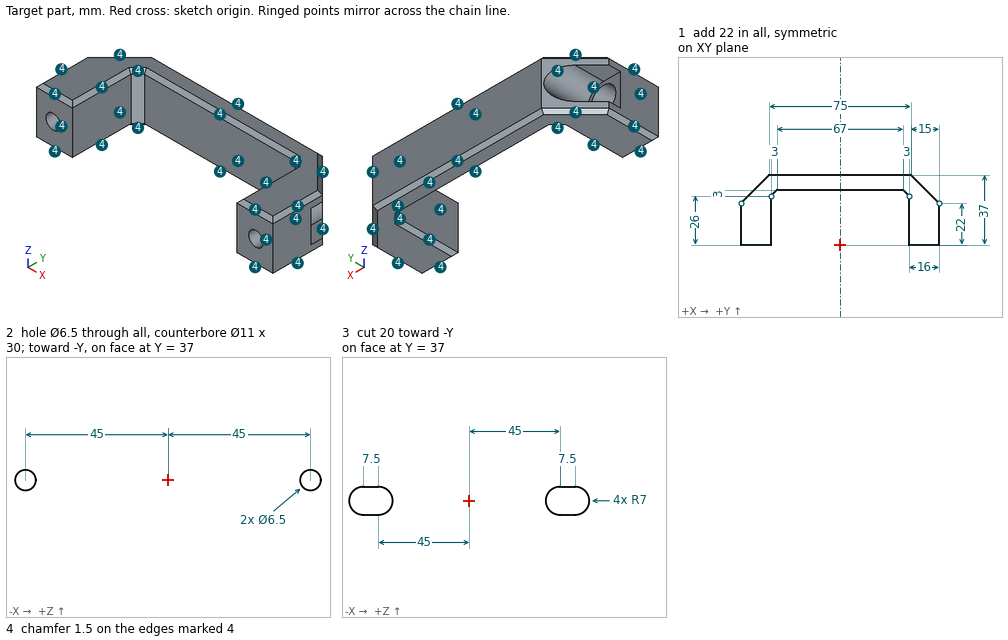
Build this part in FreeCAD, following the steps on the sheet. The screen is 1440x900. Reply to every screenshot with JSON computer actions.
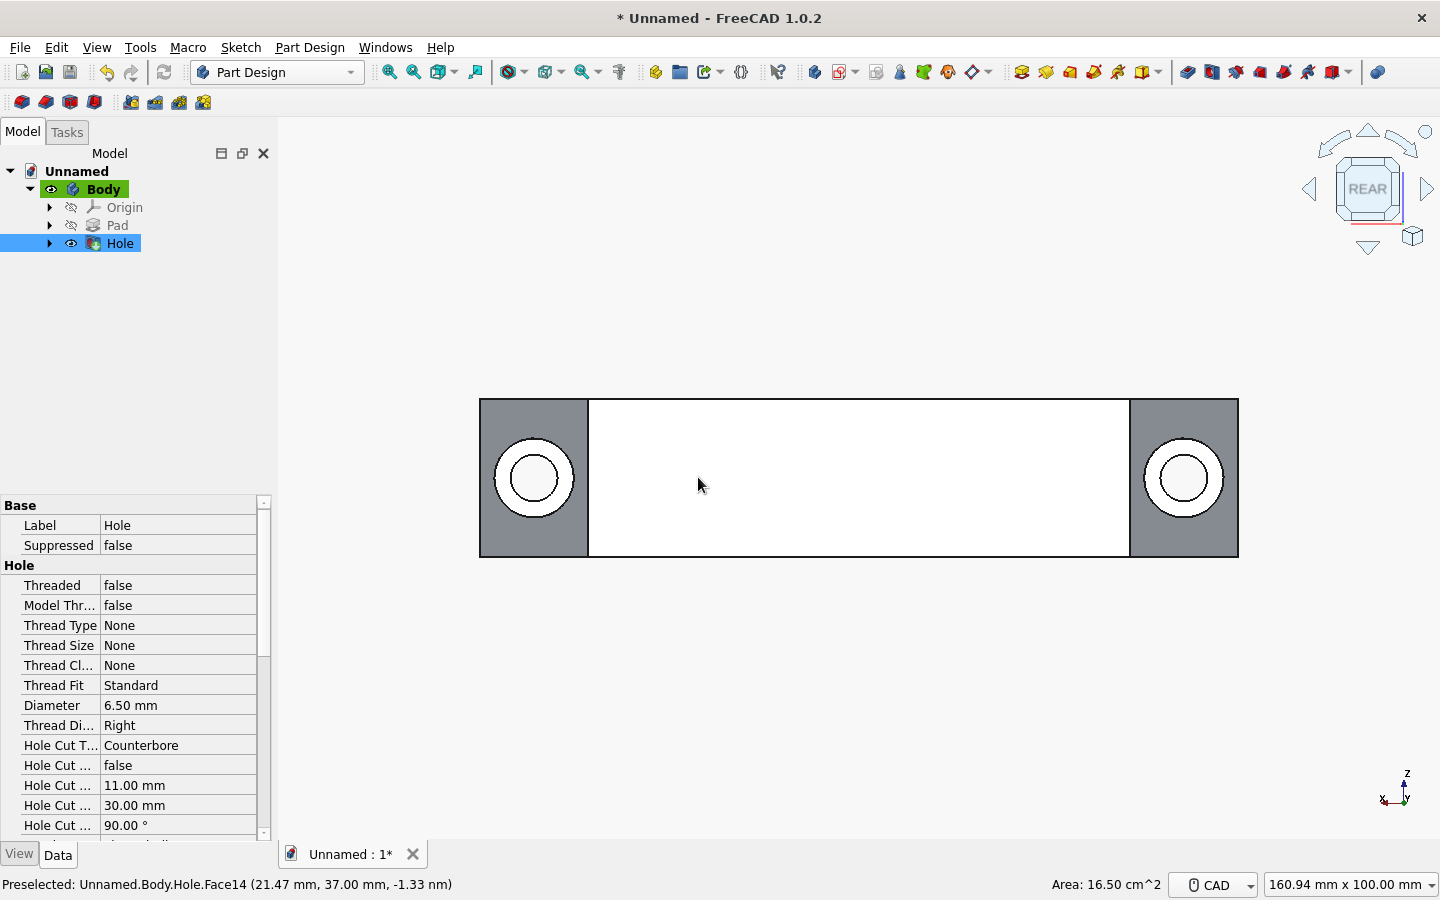
{"action": "left_click", "coordinate": [840, 72]}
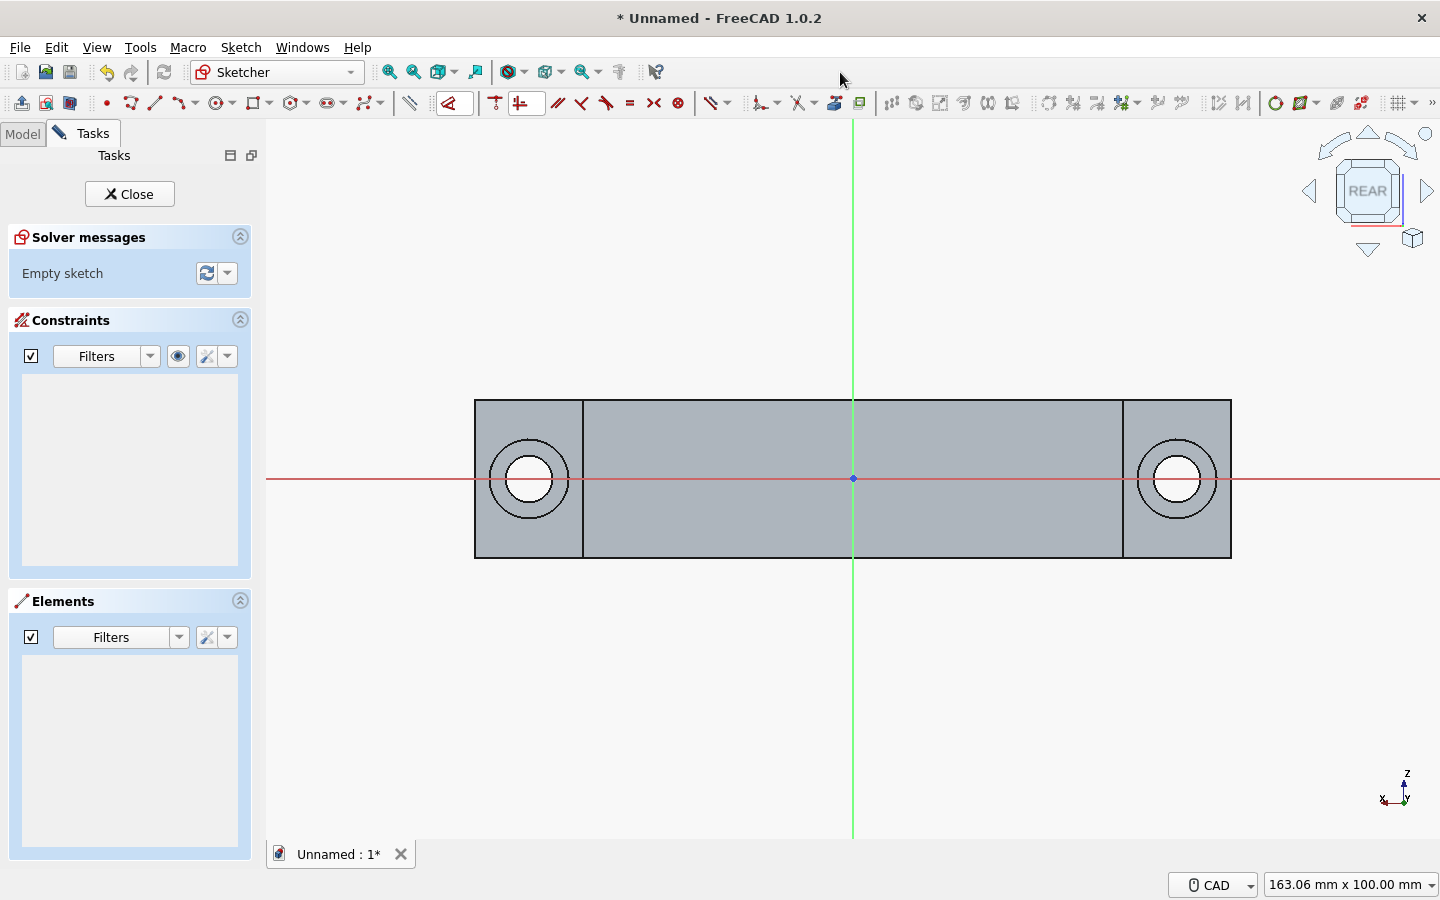
{"action": "scroll", "coordinate": [475, 479], "scroll_direction": "down", "scroll_amount": 1}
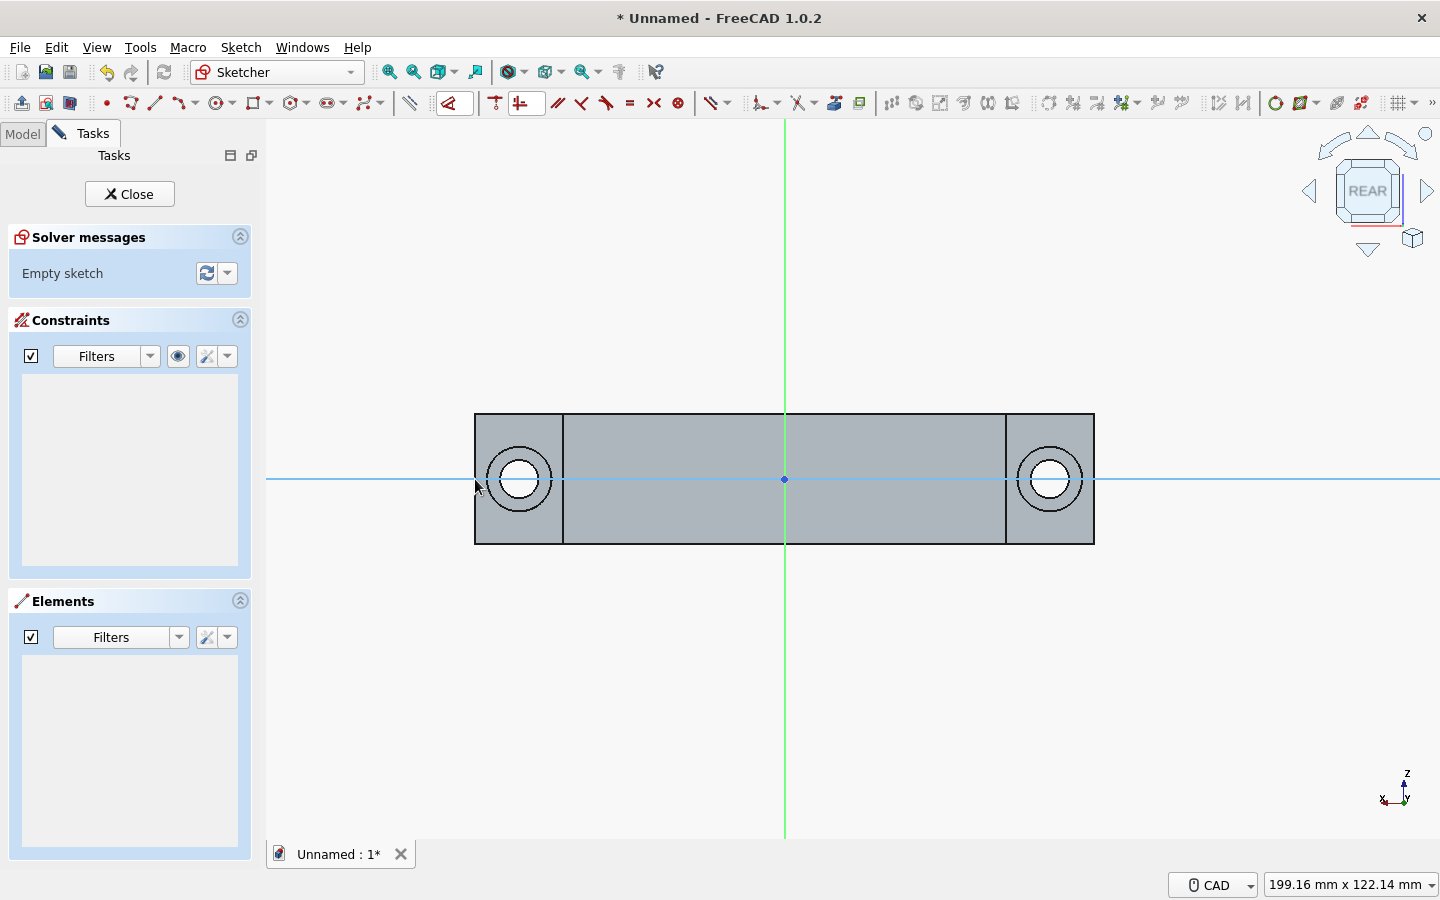
{"action": "left_click", "coordinate": [328, 104]}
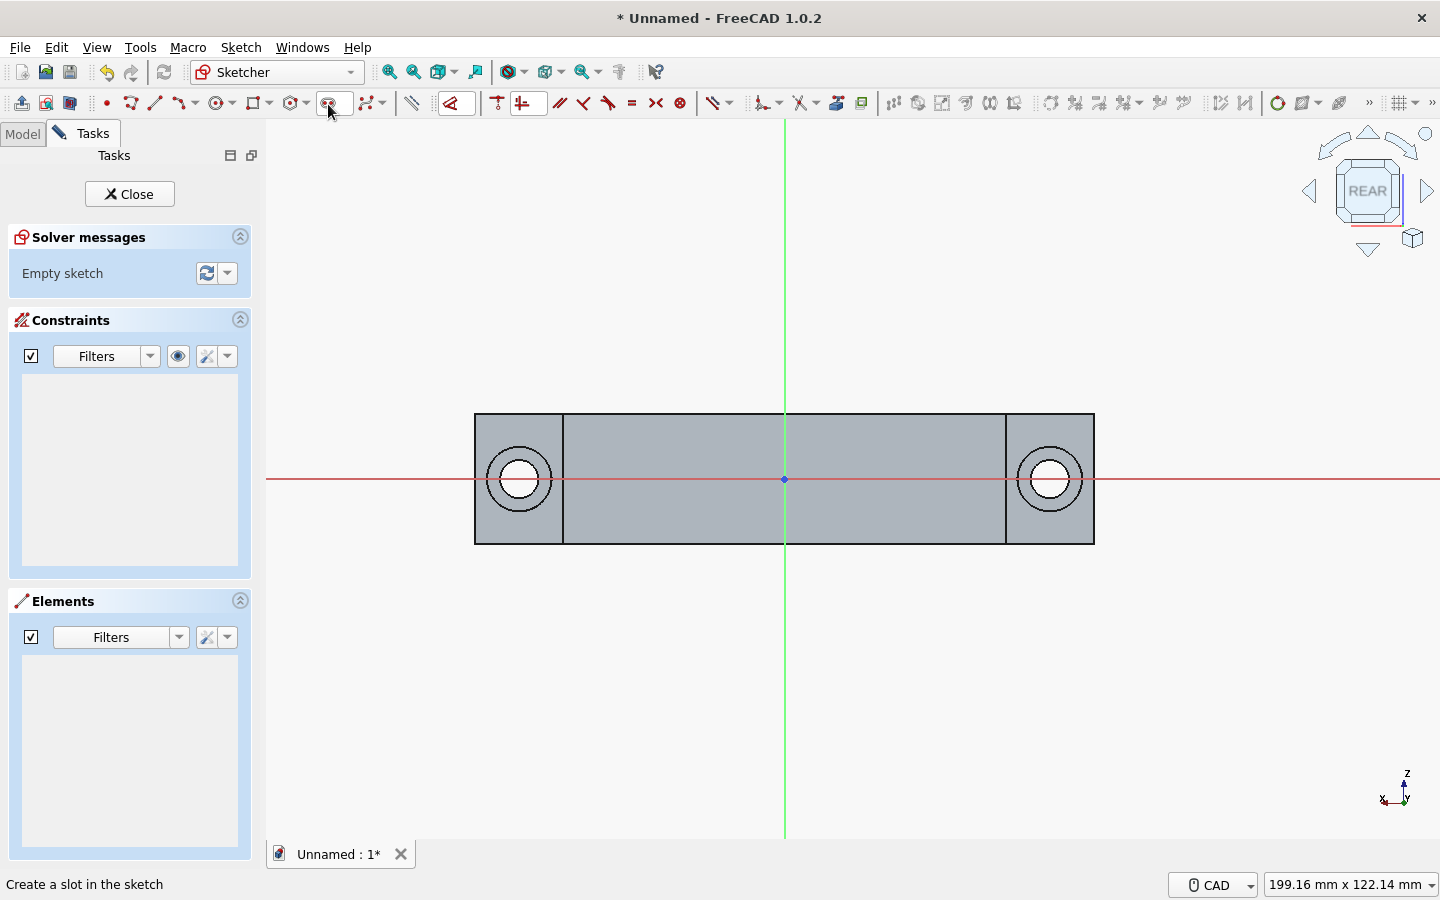
{"action": "left_click", "coordinate": [1050, 479]}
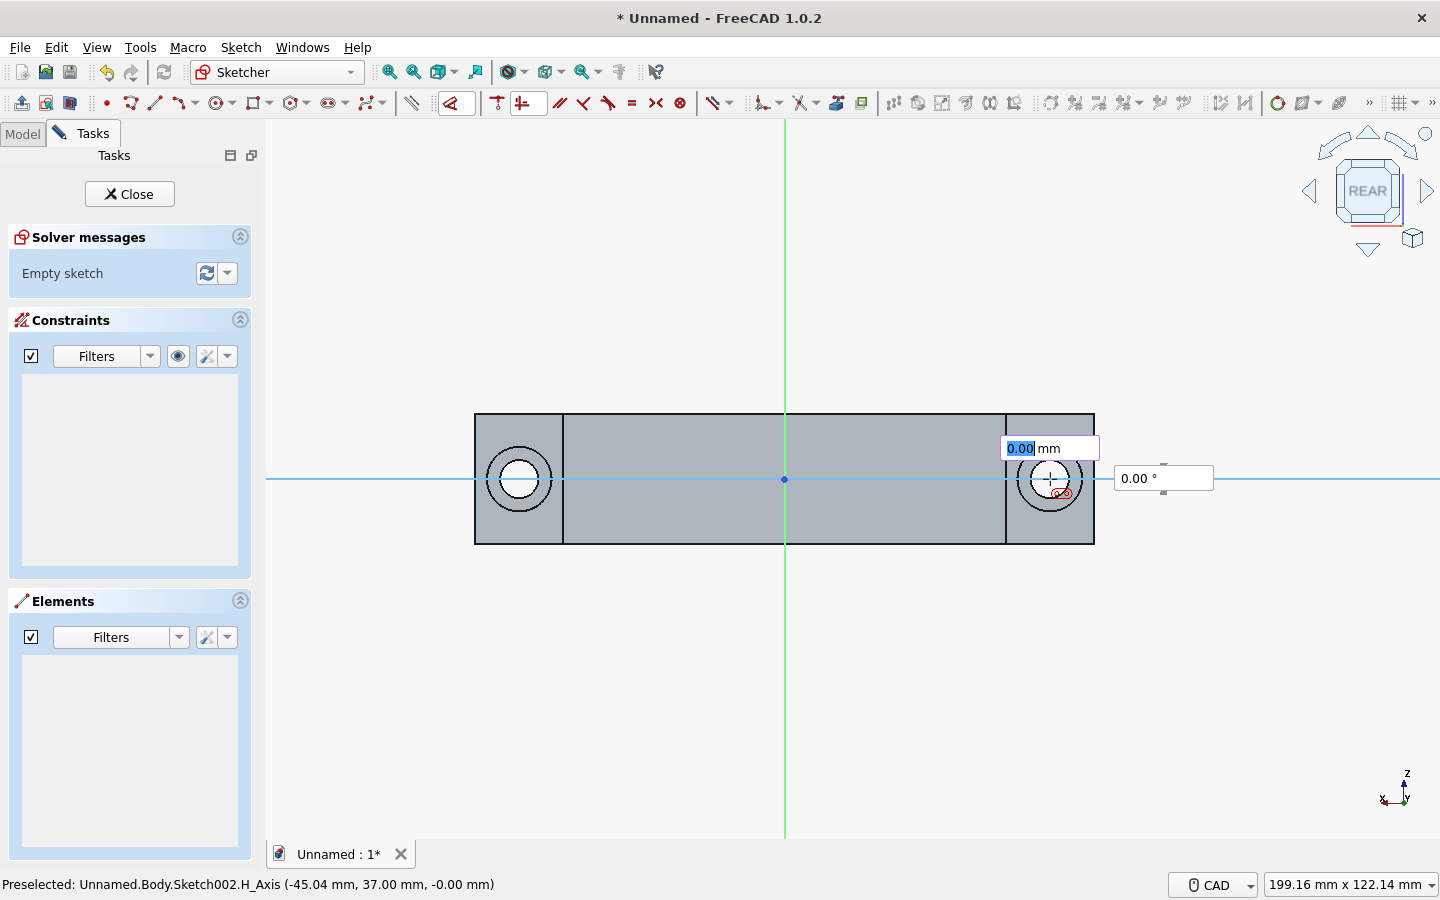
{"action": "left_click", "coordinate": [1094, 470]}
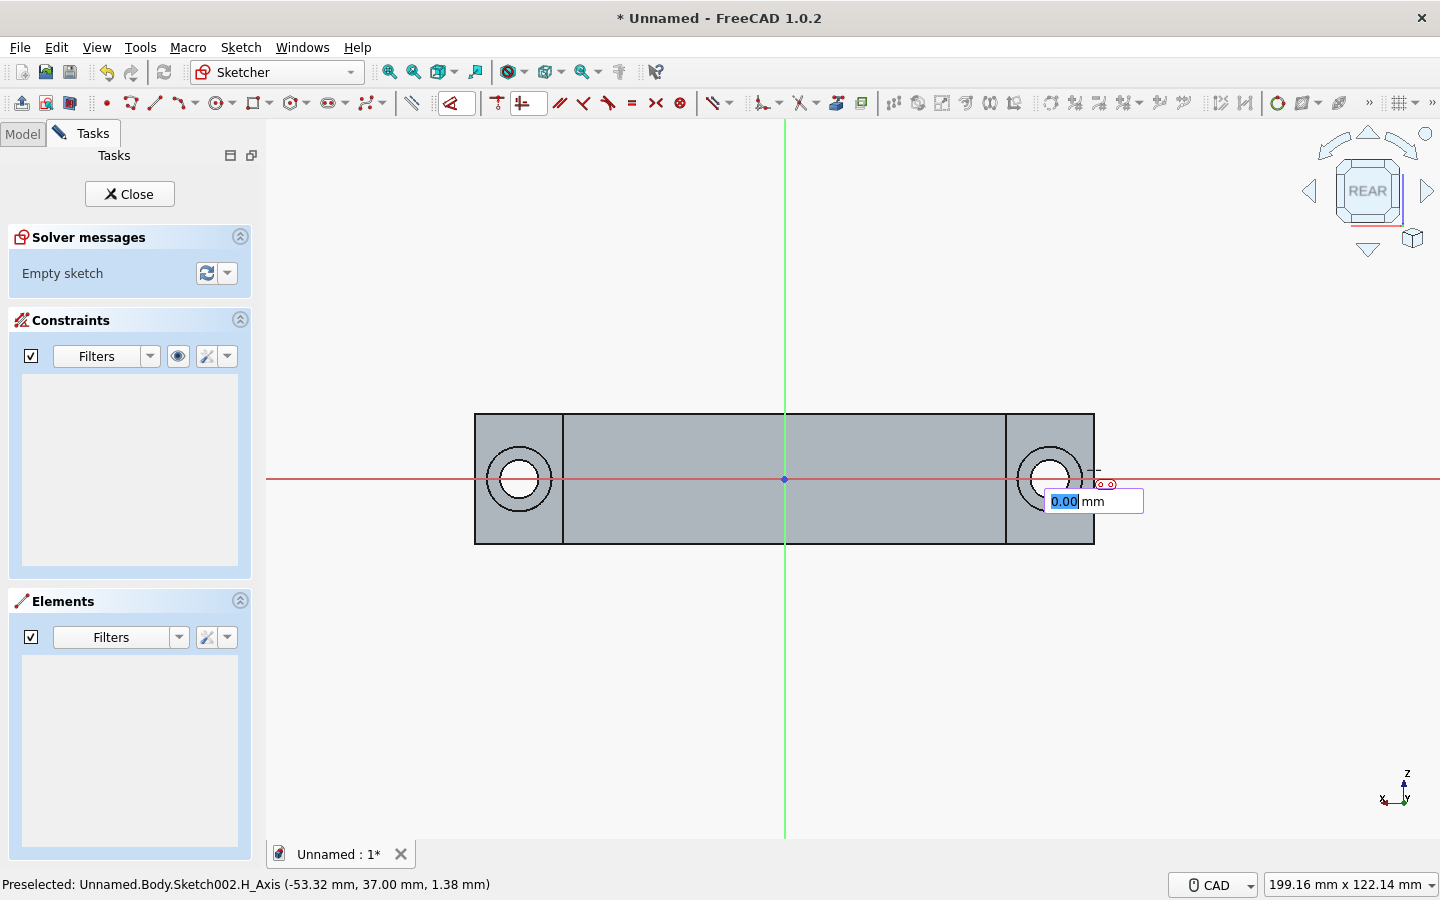
{"action": "left_click", "coordinate": [1072, 520]}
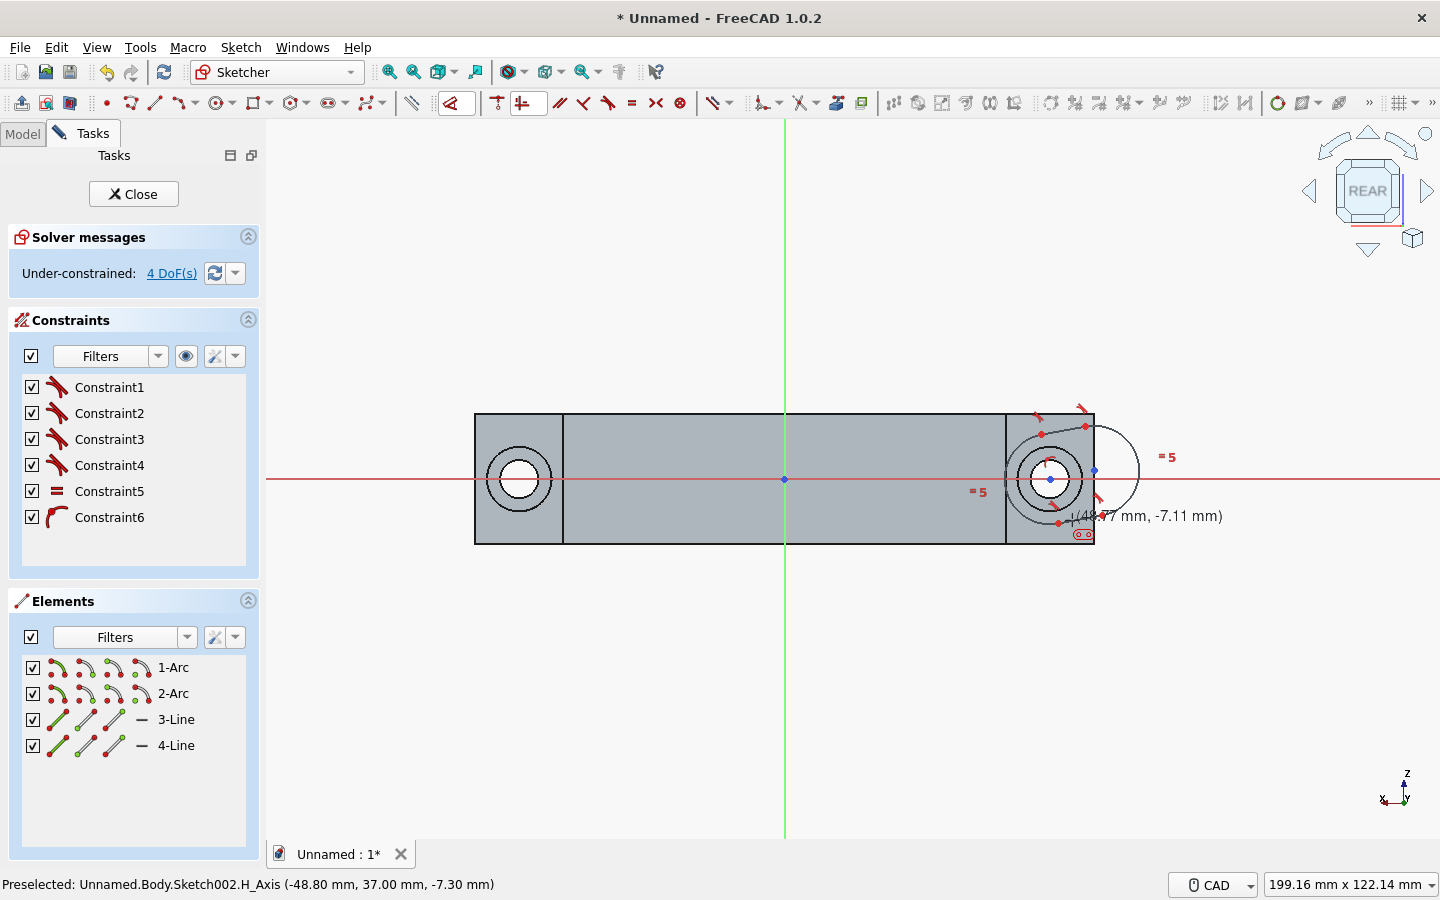
{"action": "left_click", "coordinate": [475, 479]}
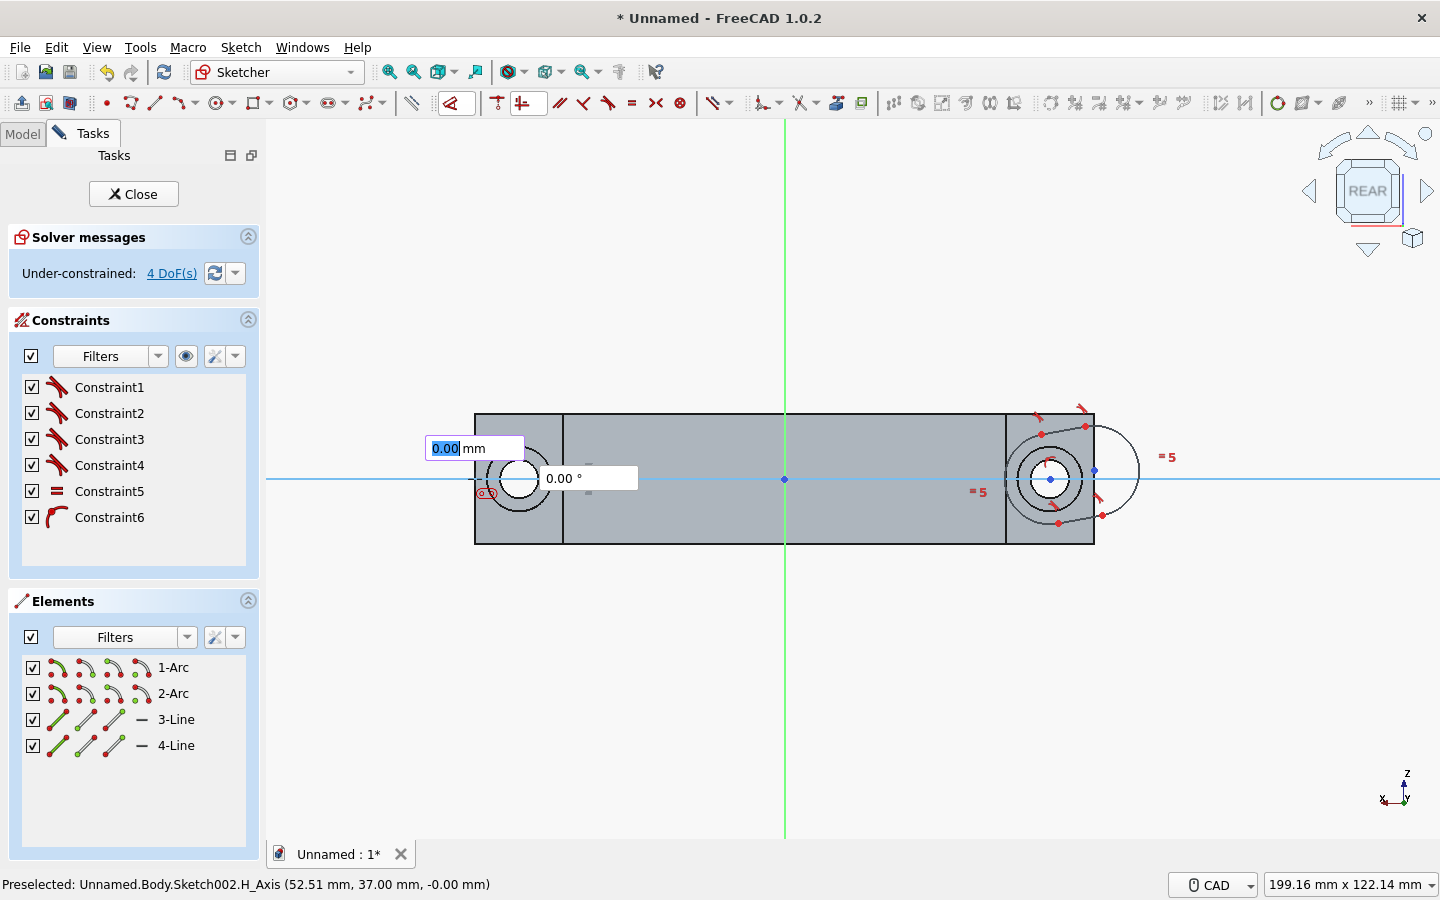
{"action": "left_click", "coordinate": [519, 470]}